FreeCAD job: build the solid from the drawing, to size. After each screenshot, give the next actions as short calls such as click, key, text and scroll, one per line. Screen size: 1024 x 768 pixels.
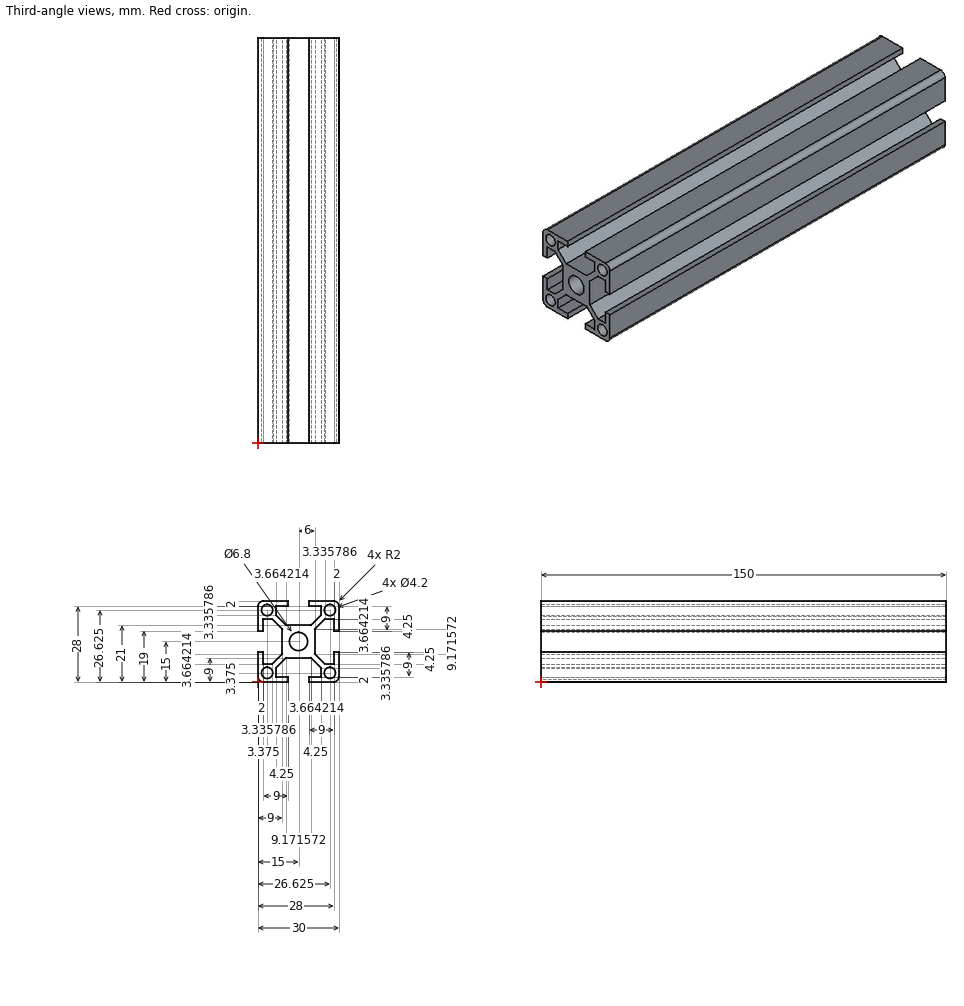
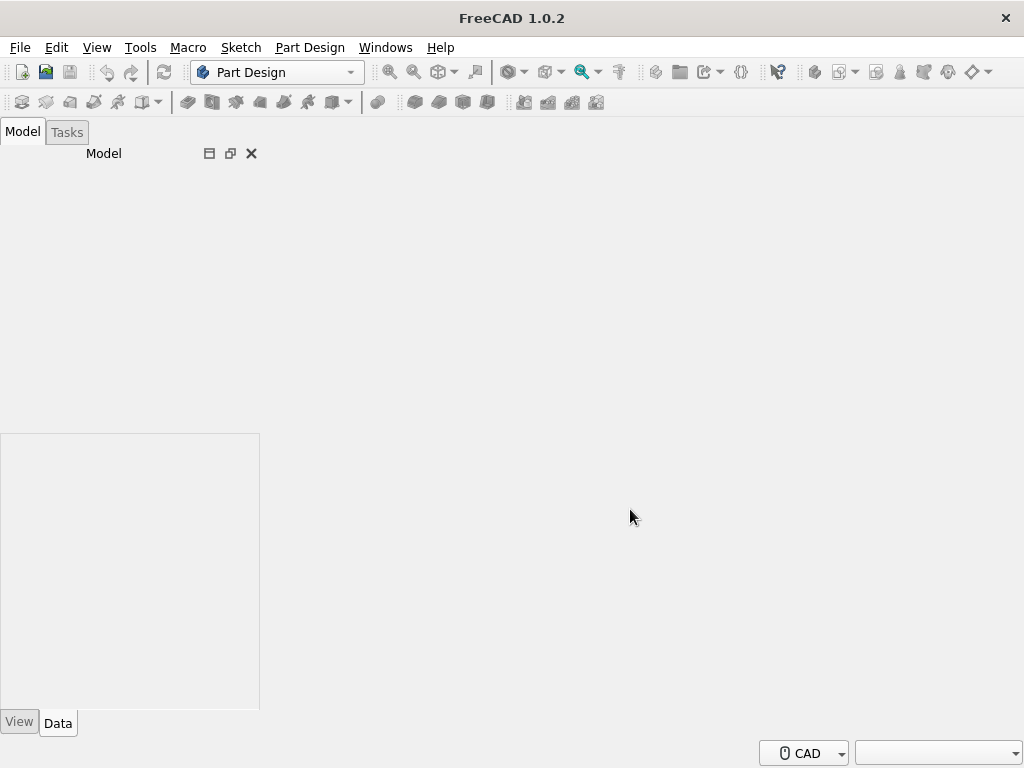
key(ctrl+n)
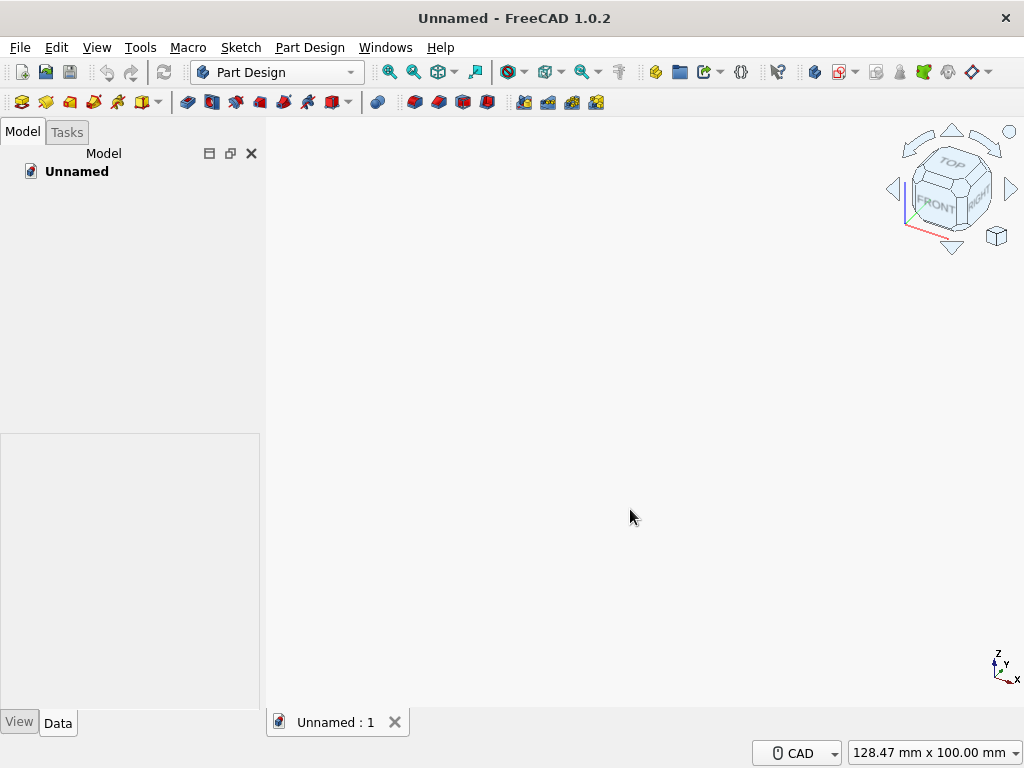
click(840, 72)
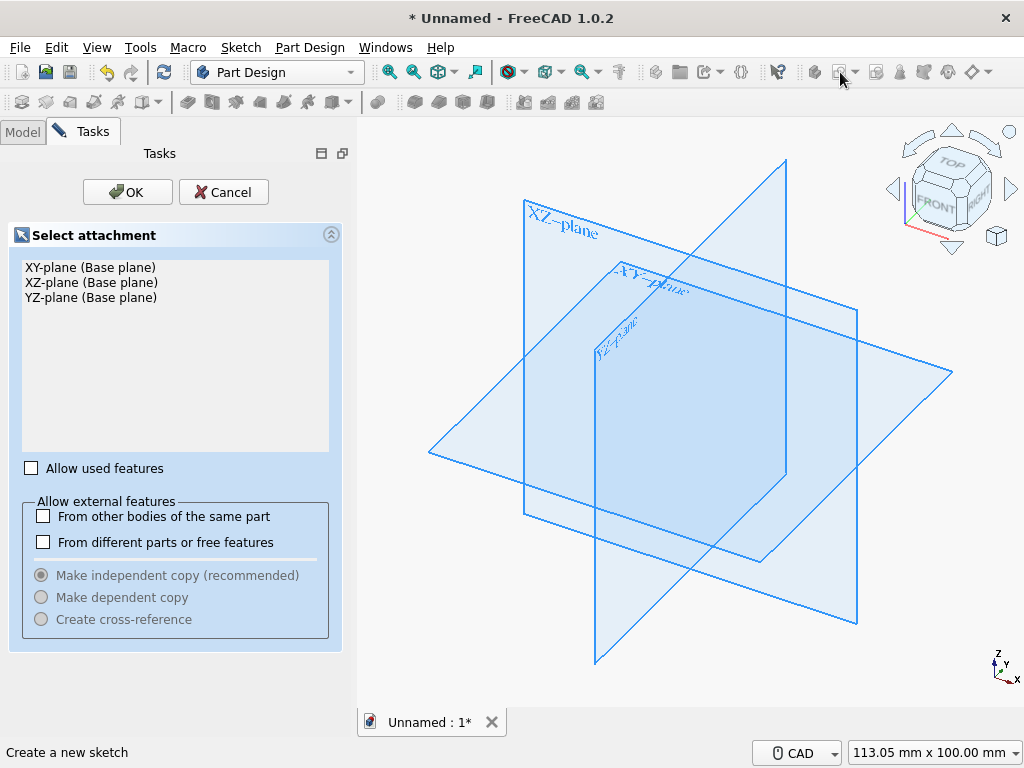
click(82, 282)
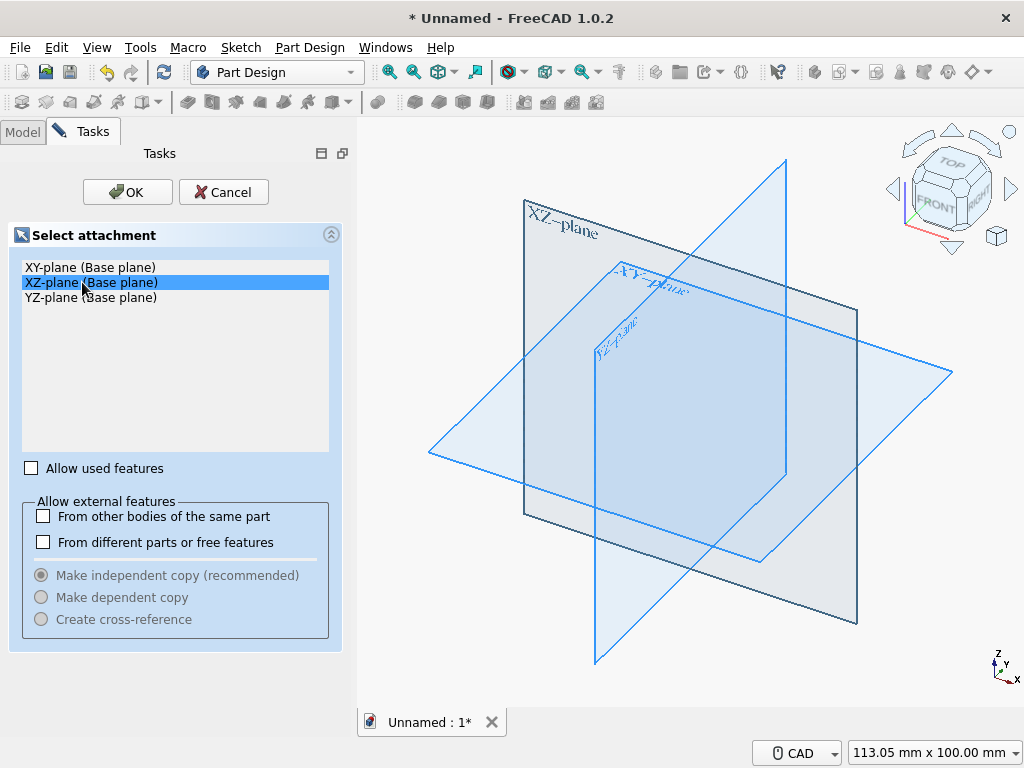
click(128, 192)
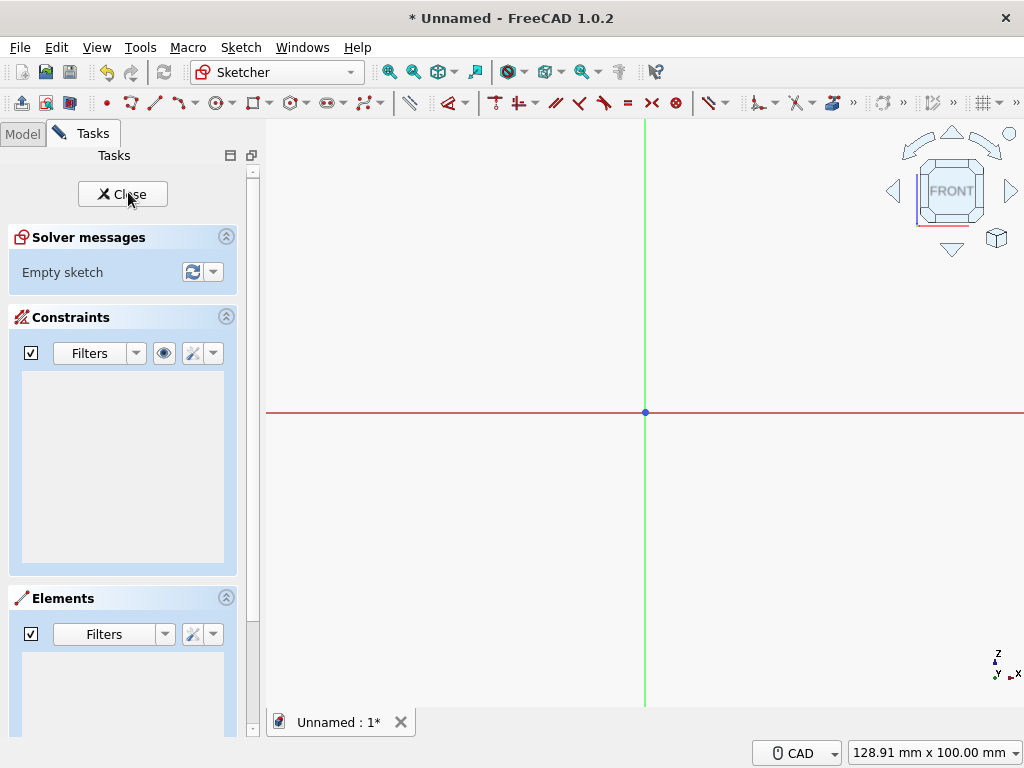
scroll(859, 253, up, 4)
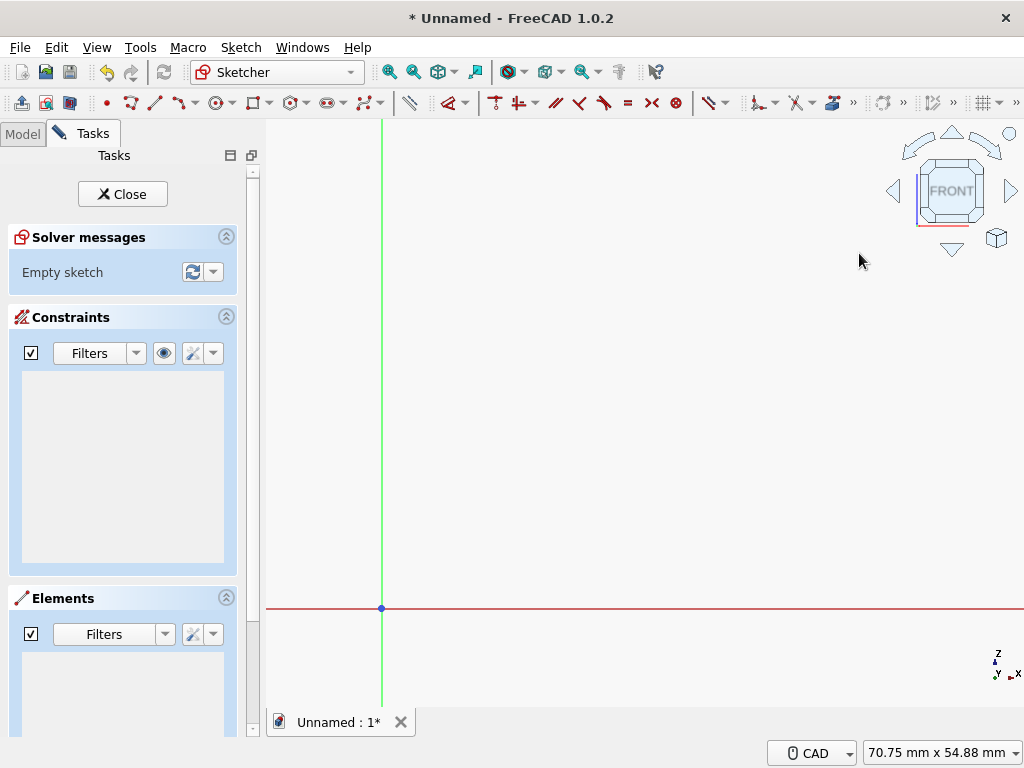
key(g)
key(m)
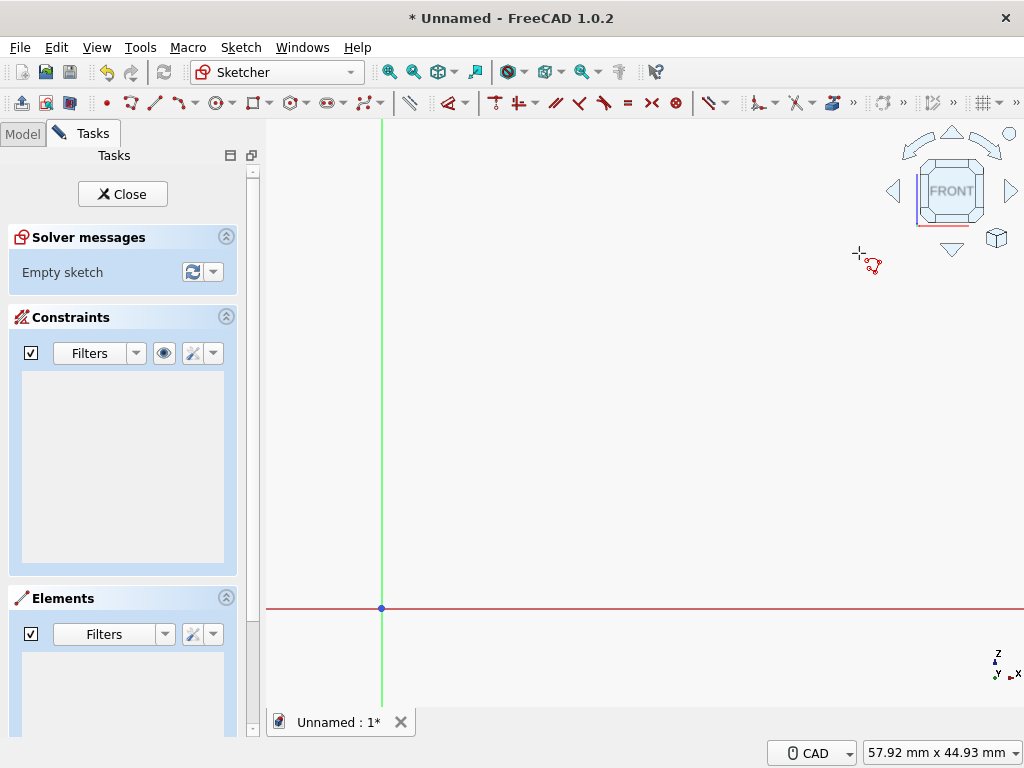
click(774, 242)
click(774, 360)
click(748, 360)
click(748, 305)
click(705, 305)
click(657, 353)
click(657, 473)
click(705, 520)
click(748, 520)
click(748, 465)
click(774, 465)
click(774, 583)
right_click(774, 583)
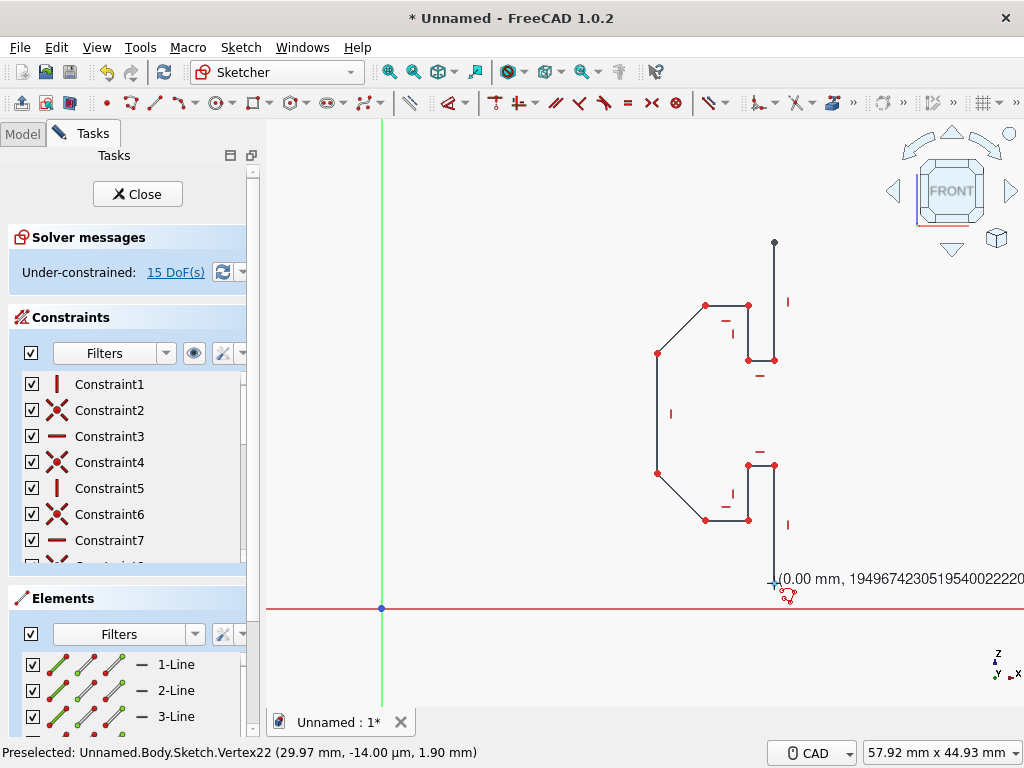
click(748, 609)
click(630, 600)
click(630, 583)
click(686, 583)
click(686, 539)
click(638, 491)
click(518, 491)
click(470, 539)
click(470, 583)
click(526, 583)
click(526, 609)
click(408, 600)
right_click(408, 600)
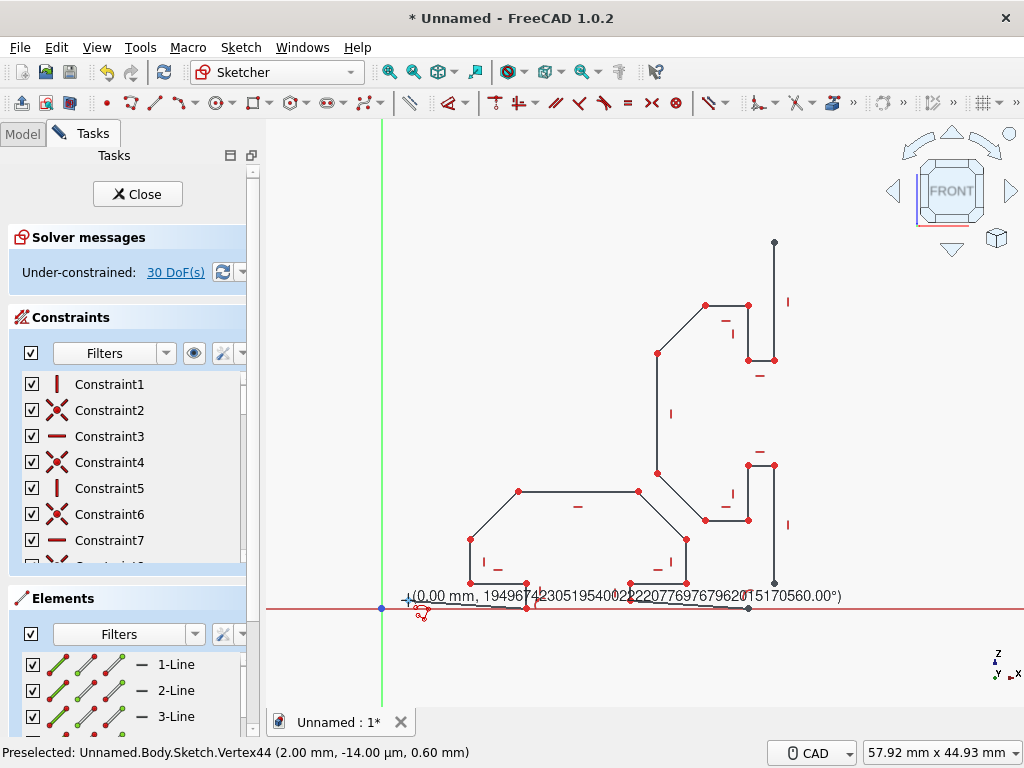
click(382, 583)
click(391, 465)
click(408, 465)
click(408, 520)
click(452, 520)
click(500, 473)
click(500, 353)
click(452, 305)
click(408, 305)
click(408, 360)
click(382, 360)
click(391, 242)
right_click(391, 242)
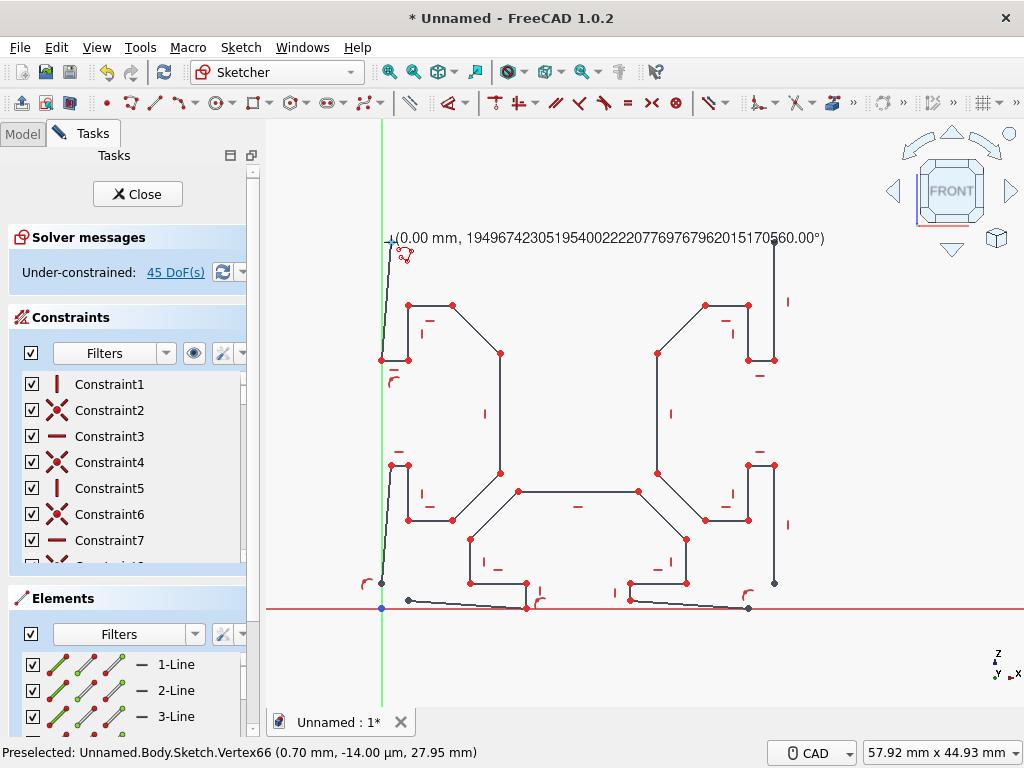
click(408, 216)
click(526, 216)
click(526, 242)
click(470, 242)
click(470, 286)
click(518, 334)
click(638, 334)
click(686, 286)
click(686, 242)
click(630, 242)
click(630, 216)
click(748, 216)
right_click(748, 216)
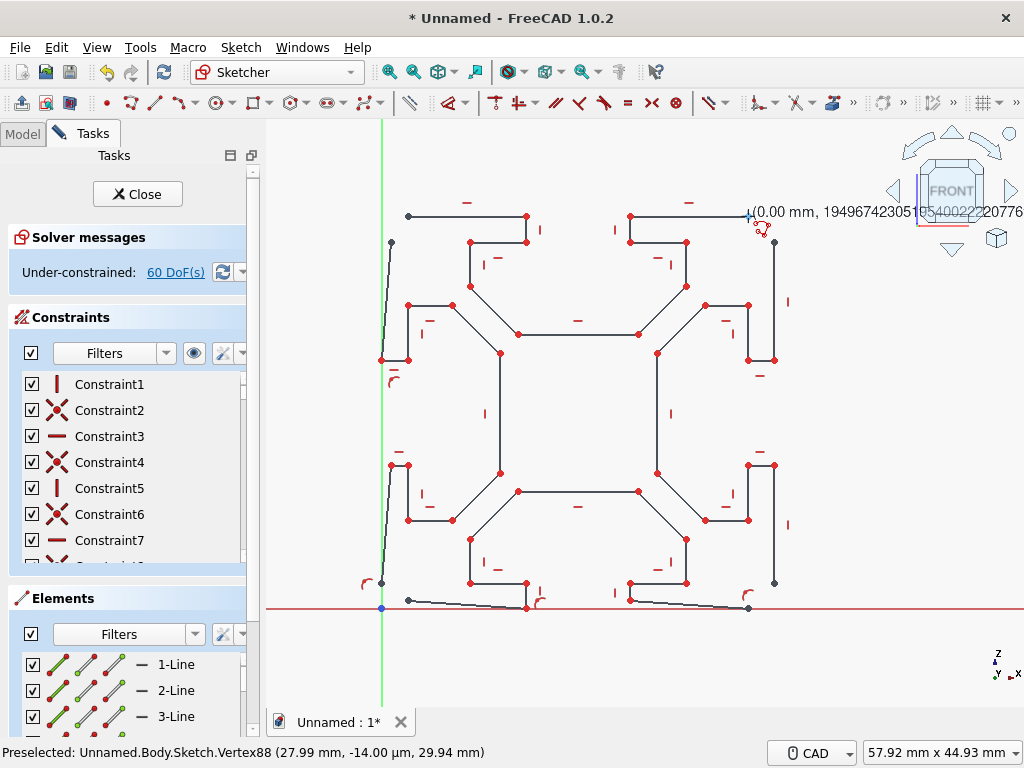
click(180, 104)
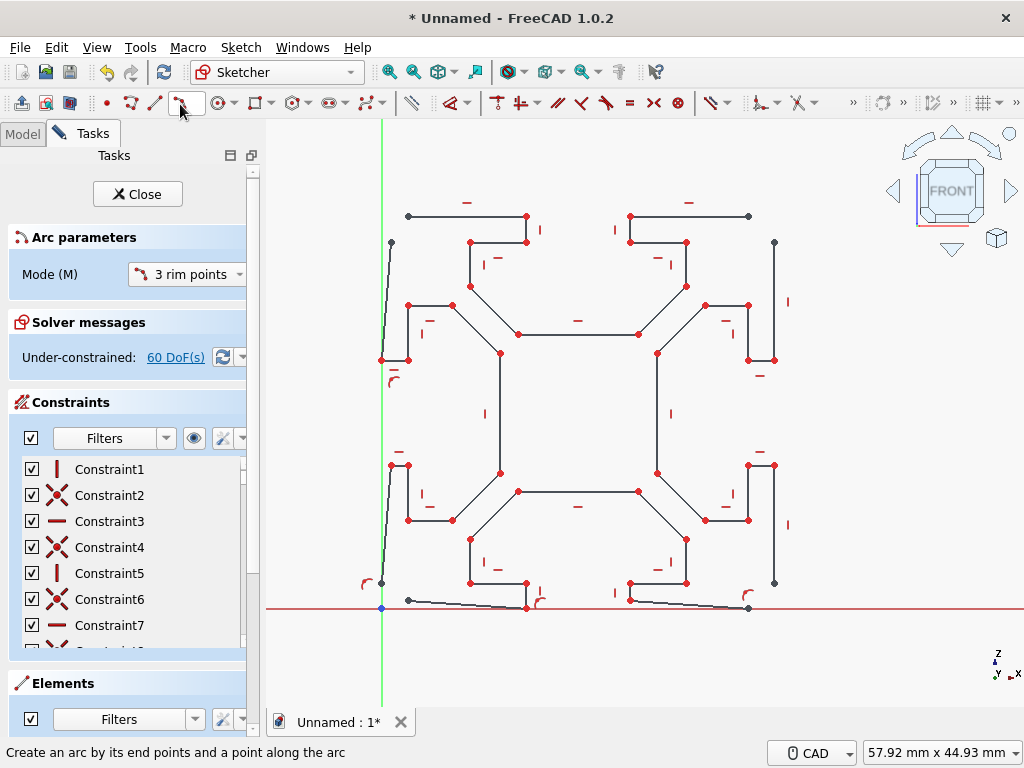
click(774, 584)
click(748, 609)